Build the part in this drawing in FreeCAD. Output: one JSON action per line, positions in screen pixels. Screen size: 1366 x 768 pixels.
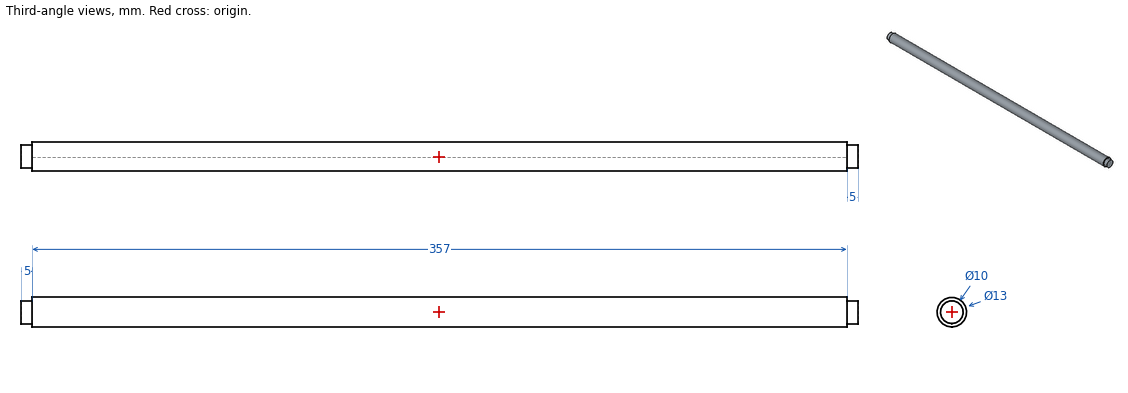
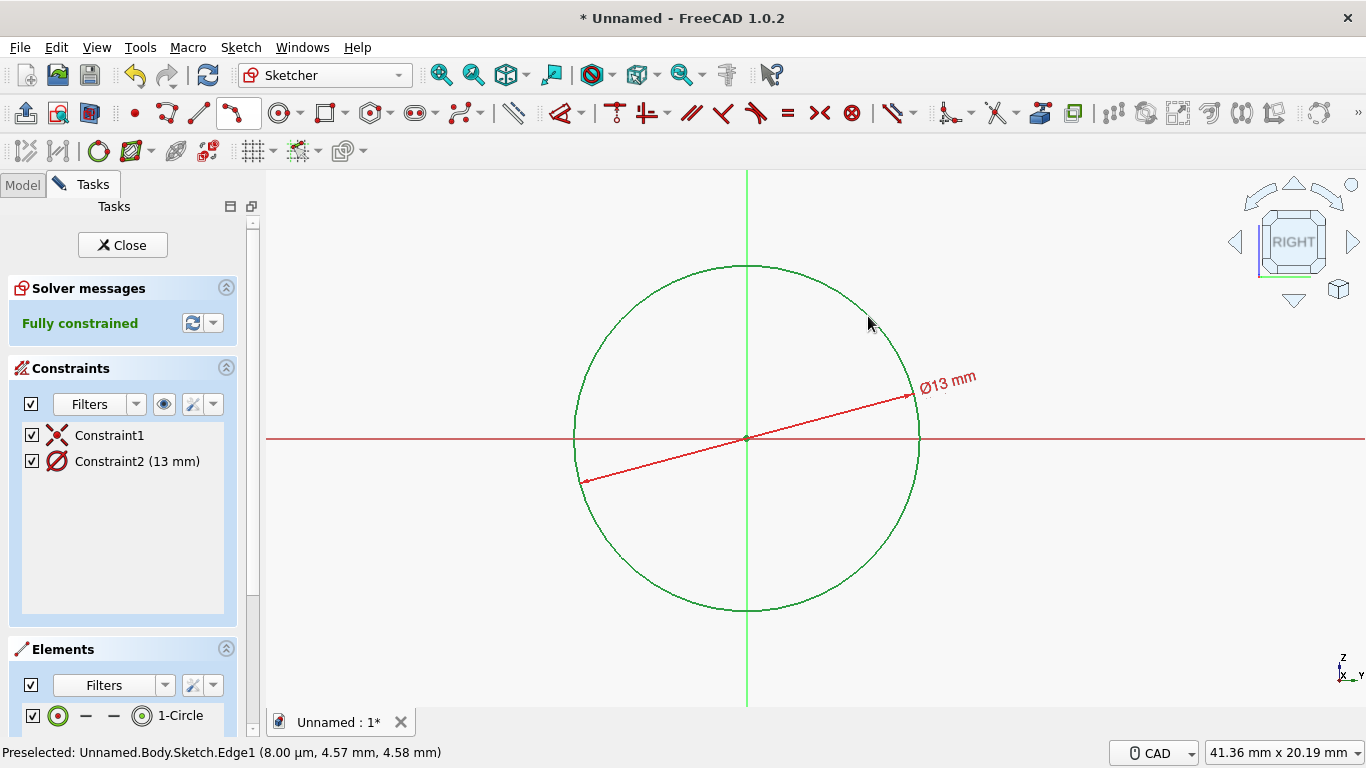
{"action": "left_click", "coordinate": [123, 245]}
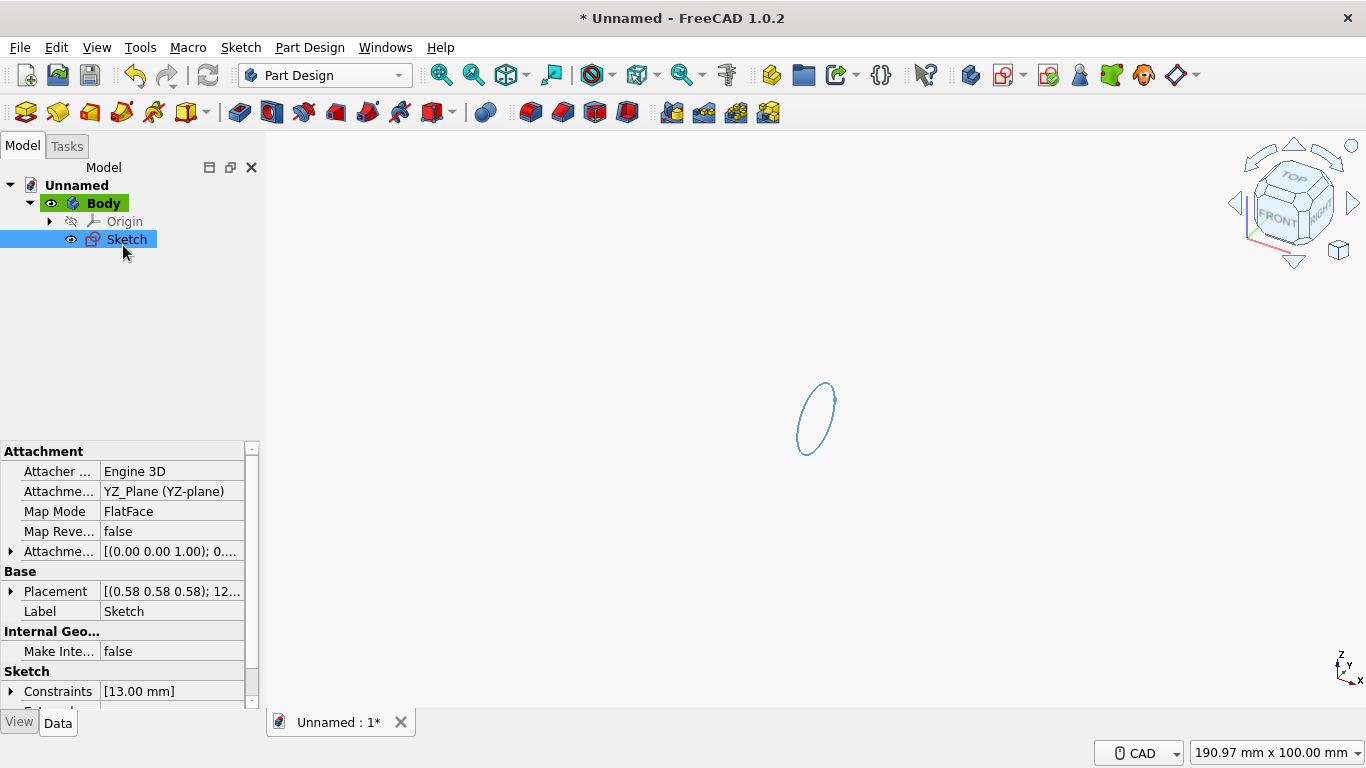
{"action": "left_click", "coordinate": [26, 112]}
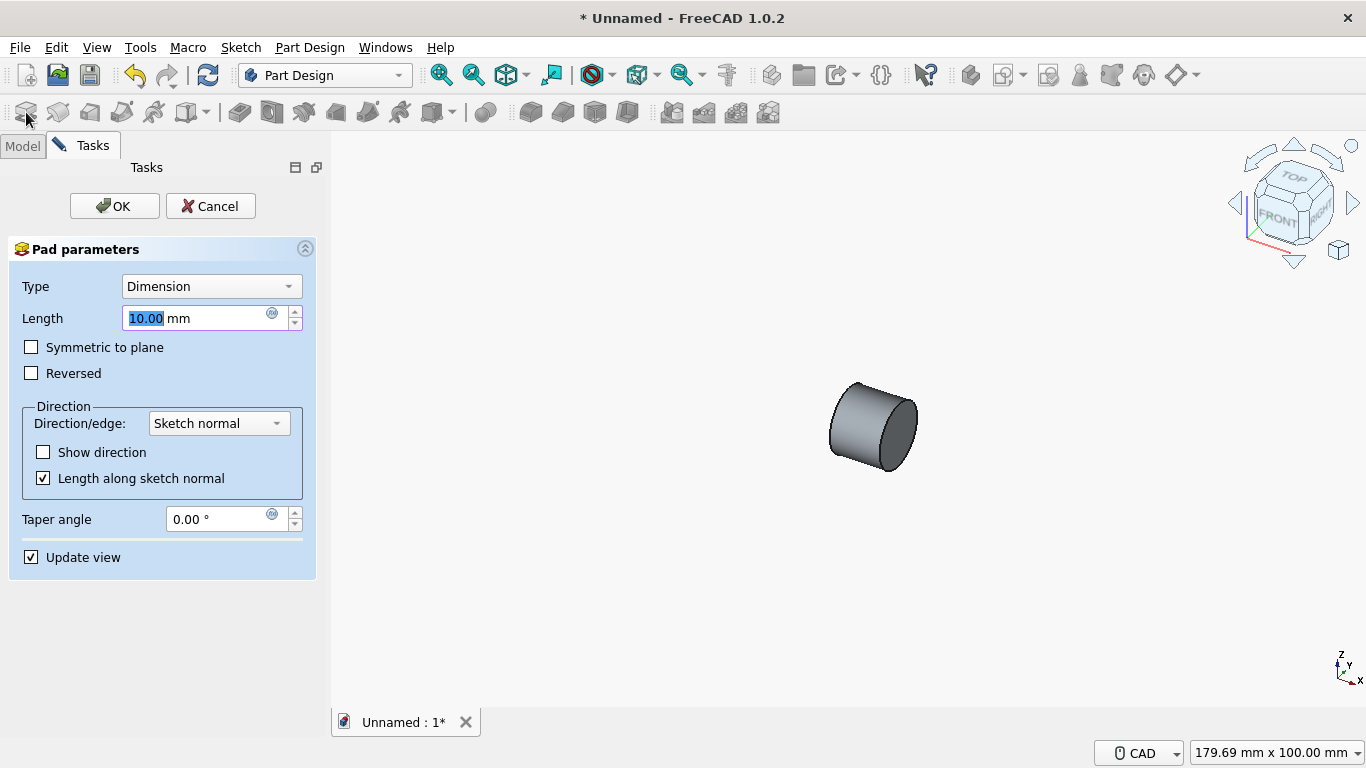
{"action": "type", "text": "357"}
{"action": "key", "text": "Tab"}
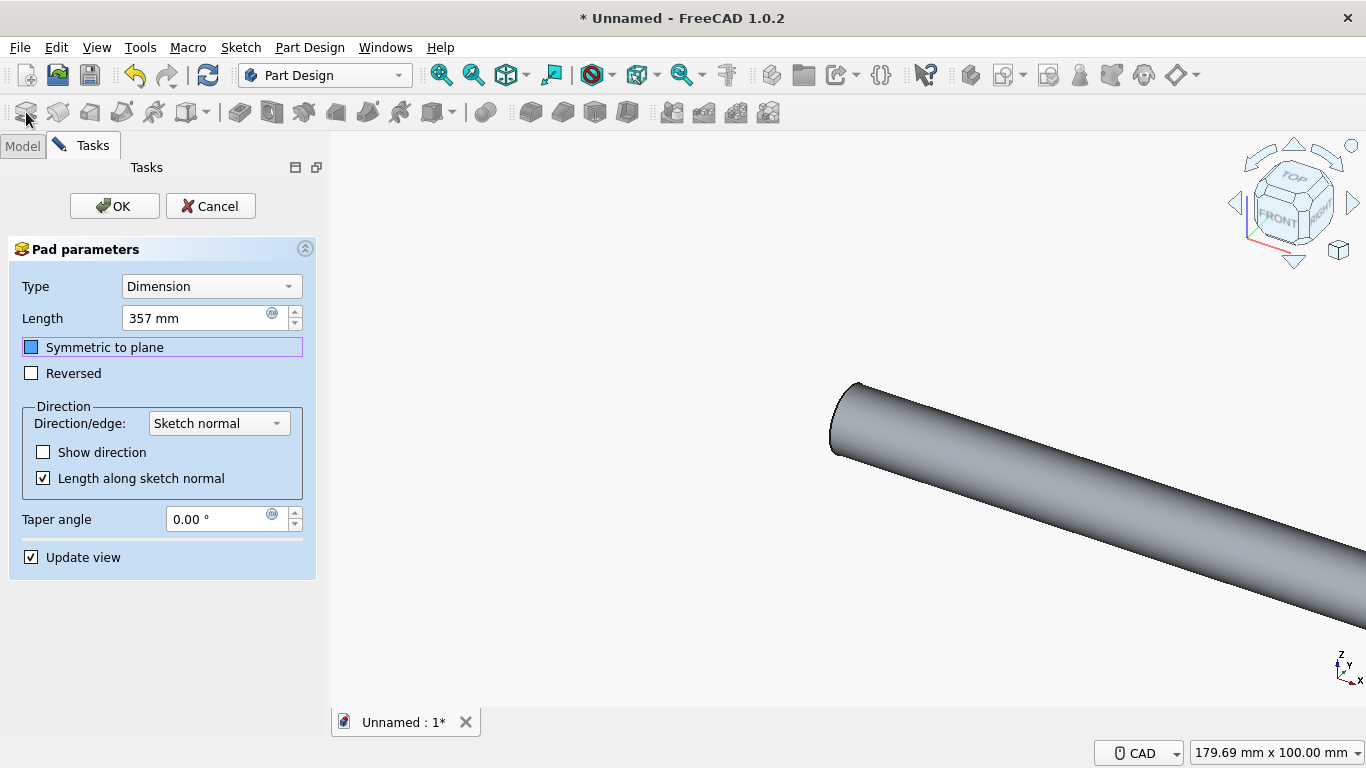
{"action": "left_click", "coordinate": [30, 347]}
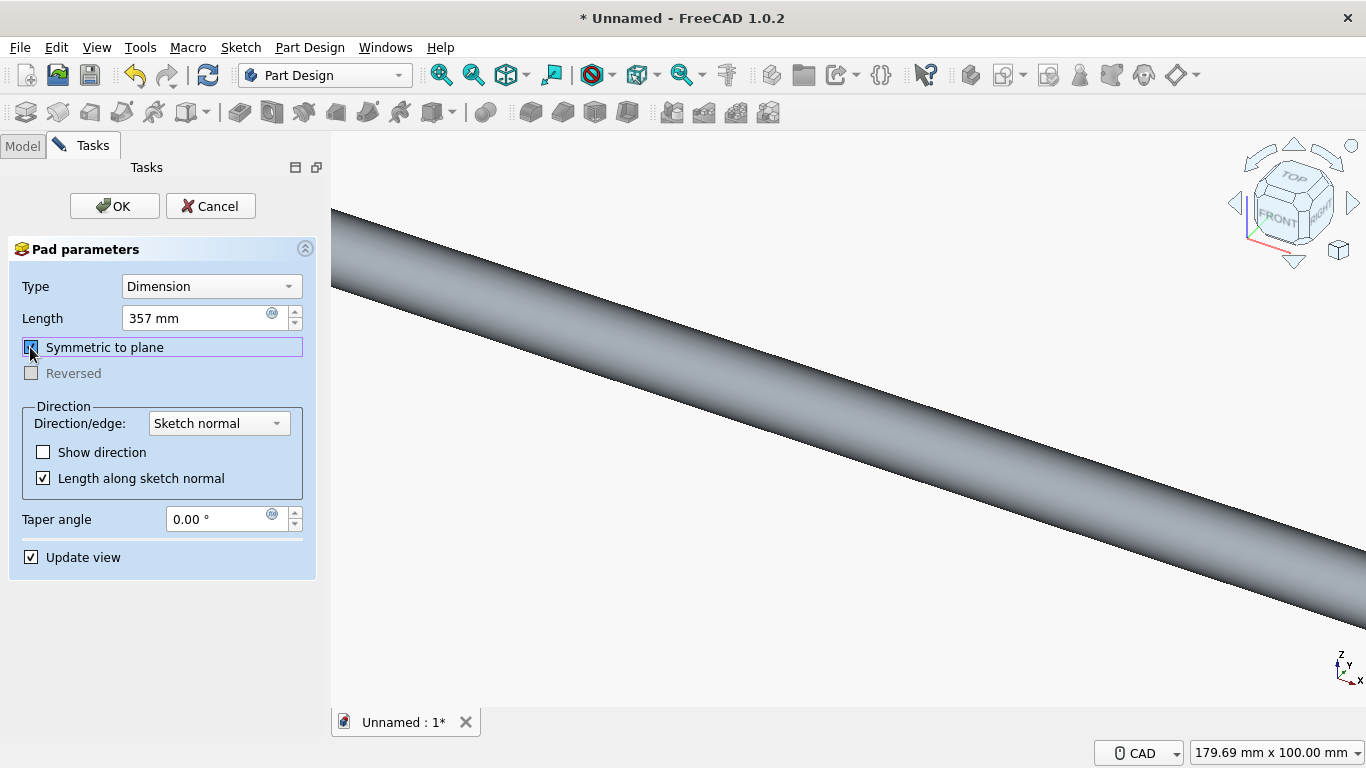
{"action": "left_click", "coordinate": [115, 206]}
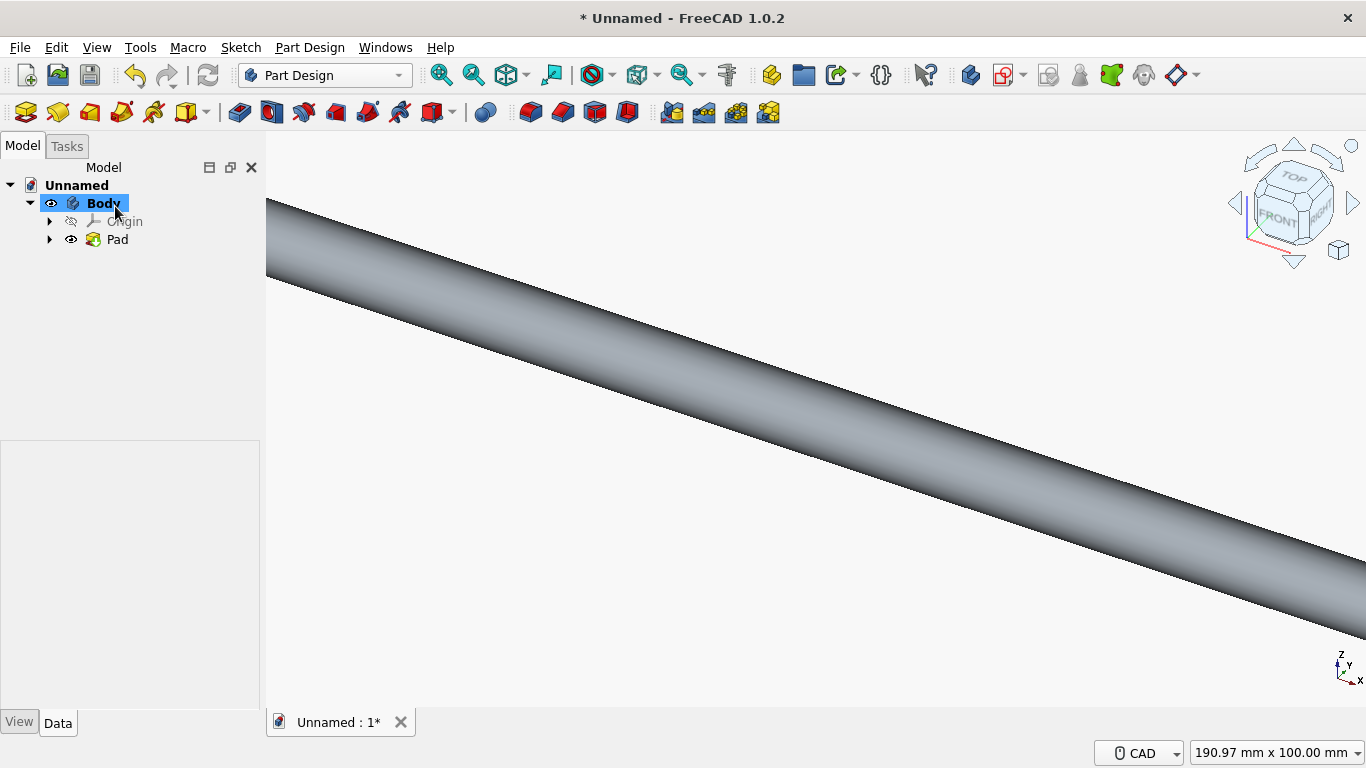
{"action": "left_click", "coordinate": [442, 76]}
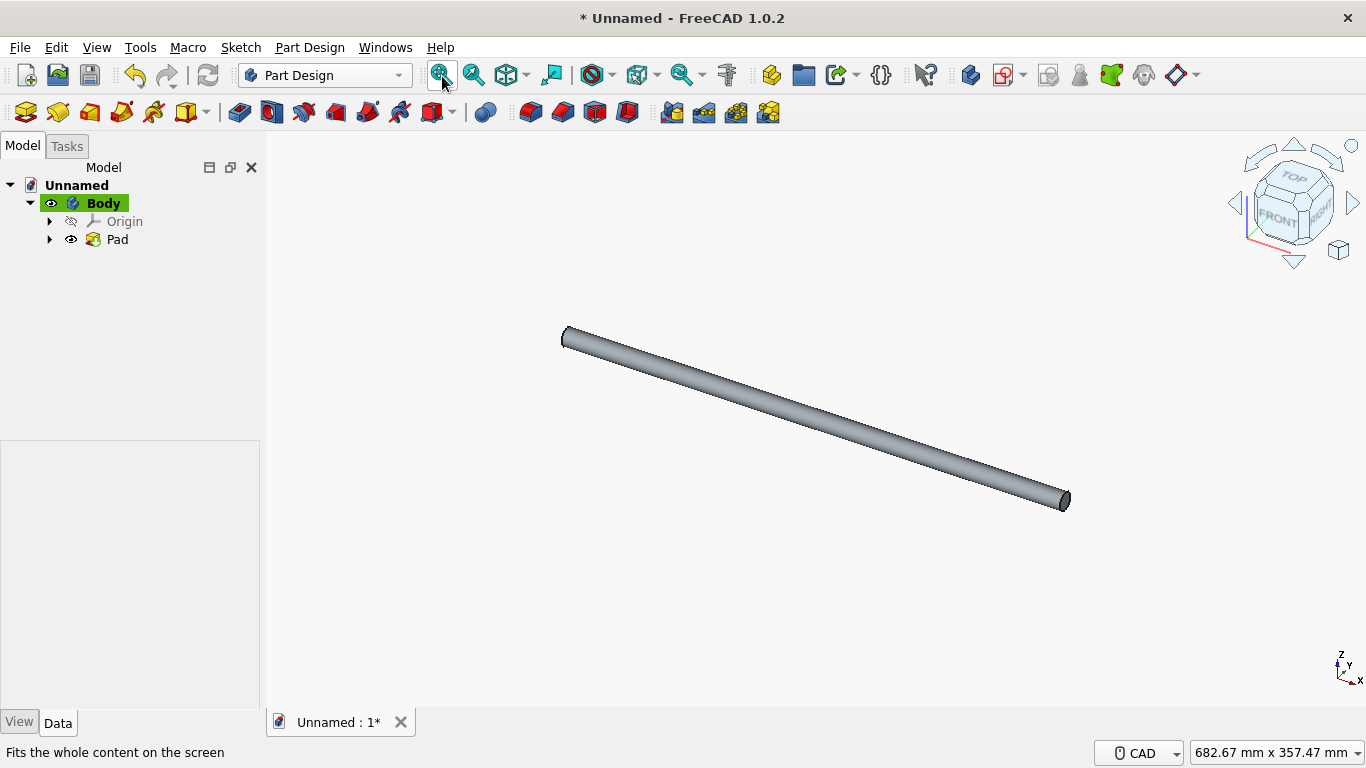
{"action": "key", "text": "0"}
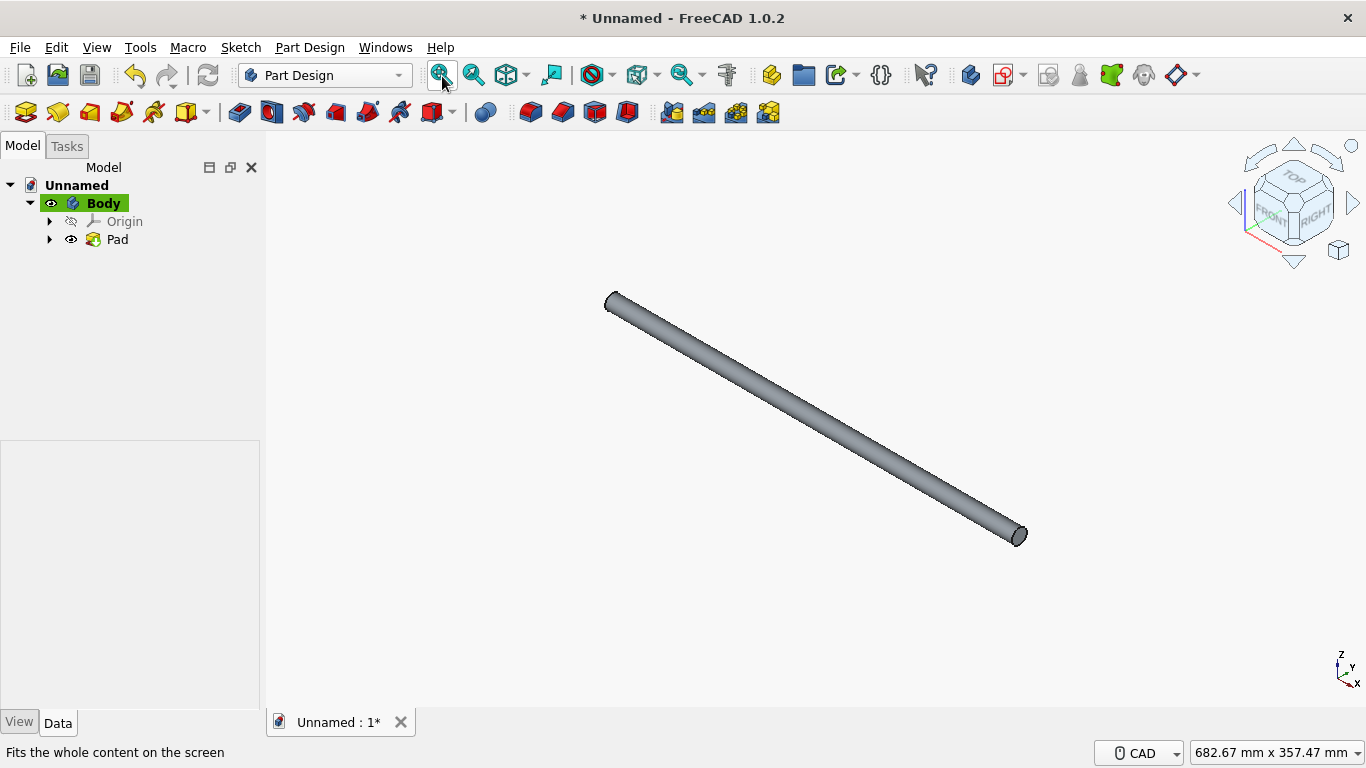
{"action": "key", "text": "3"}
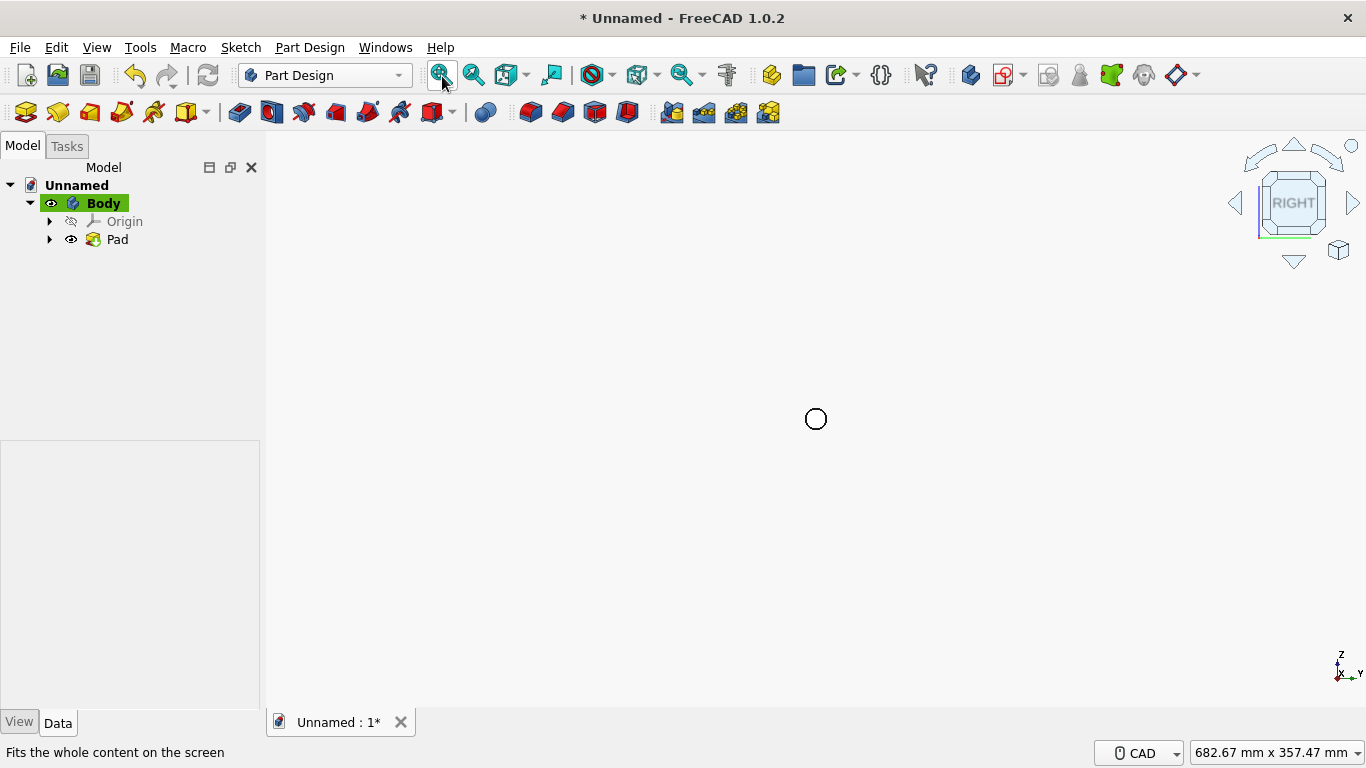
{"action": "left_click", "coordinate": [442, 76]}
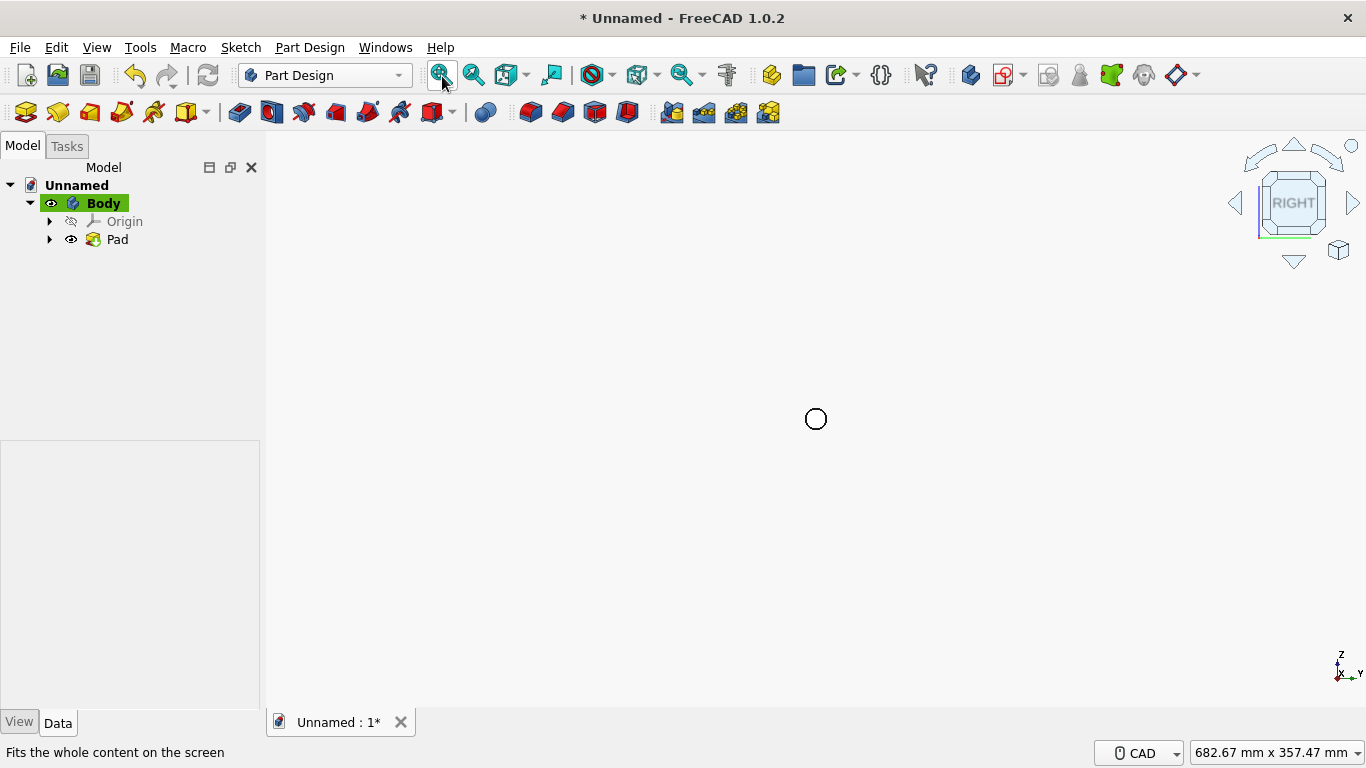
{"action": "left_click", "coordinate": [816, 418]}